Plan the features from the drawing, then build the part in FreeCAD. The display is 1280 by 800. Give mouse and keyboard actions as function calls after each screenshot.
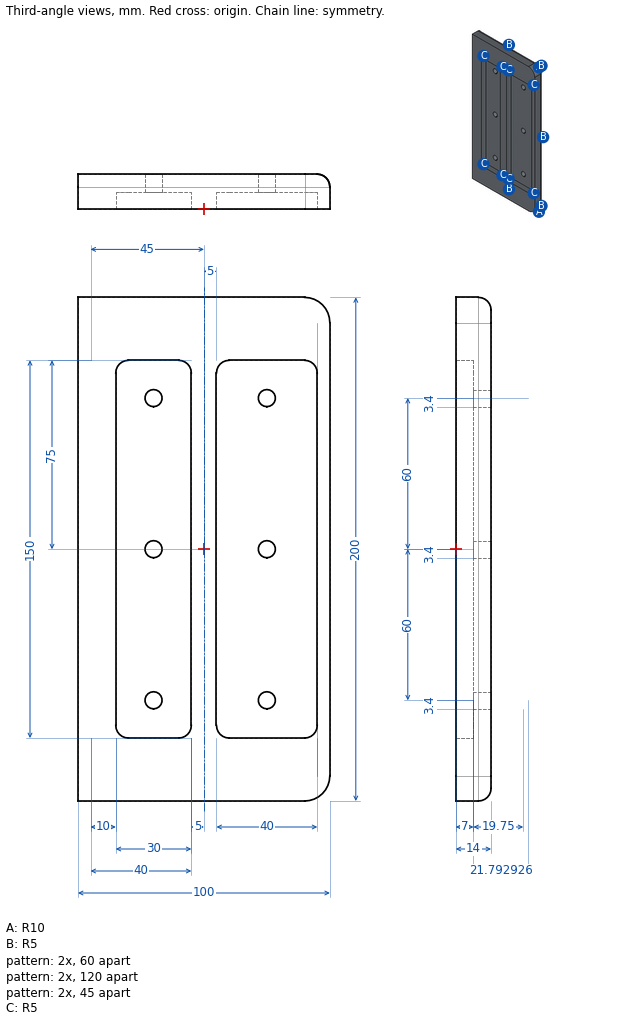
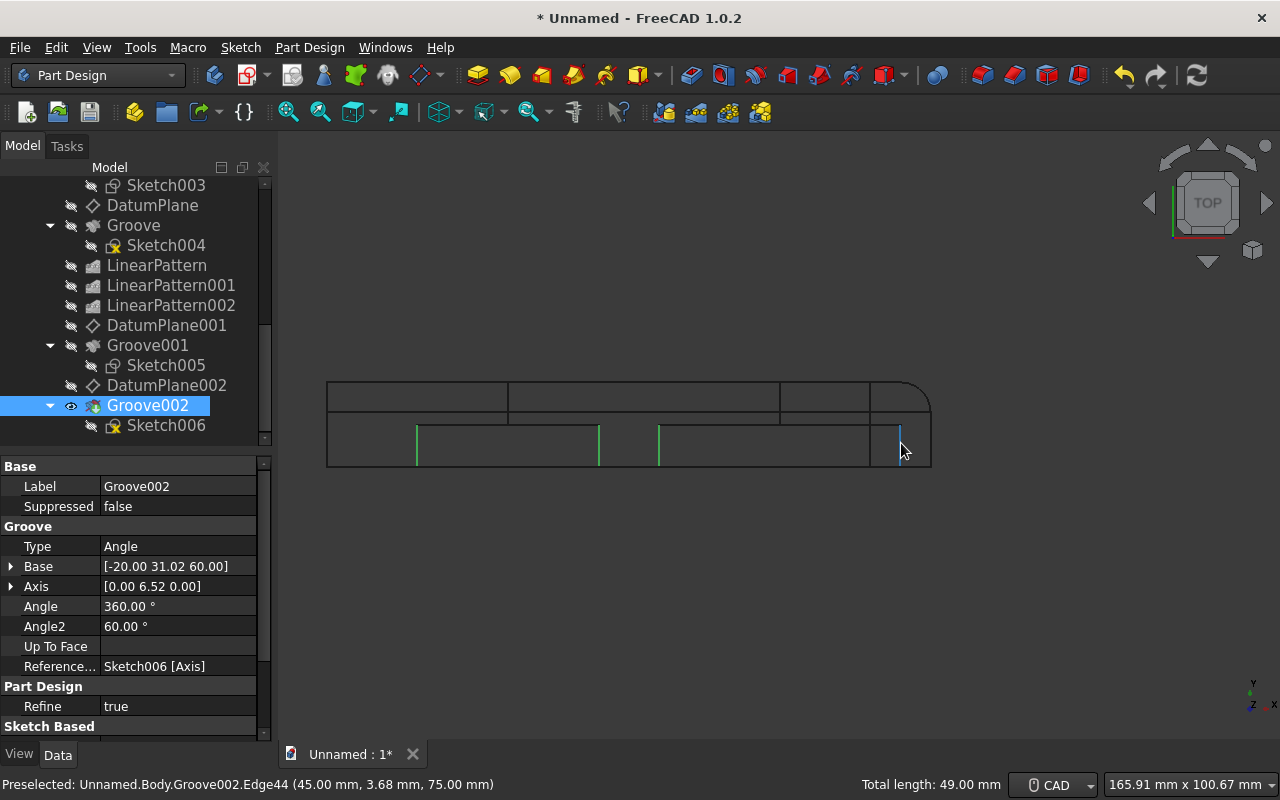
key(v)
key(f)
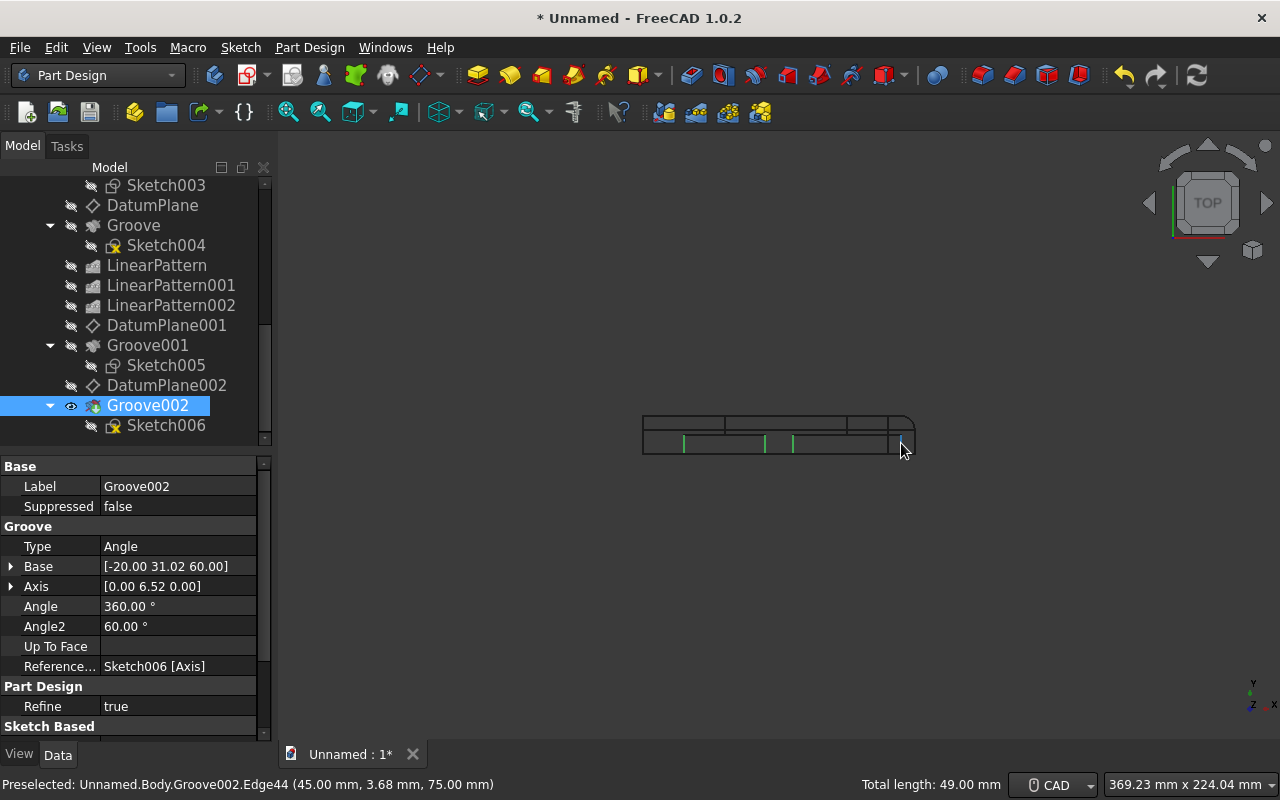
key(1)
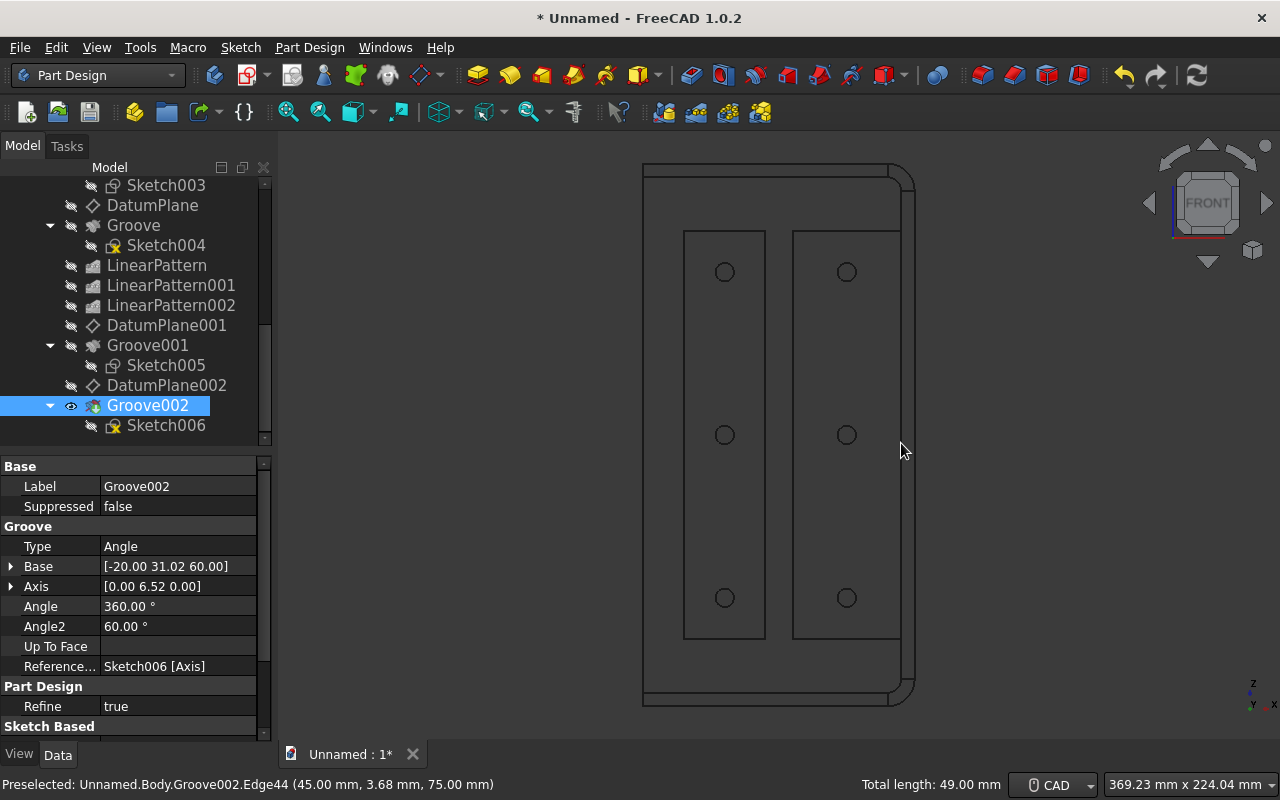
scroll(901, 638, up, 4)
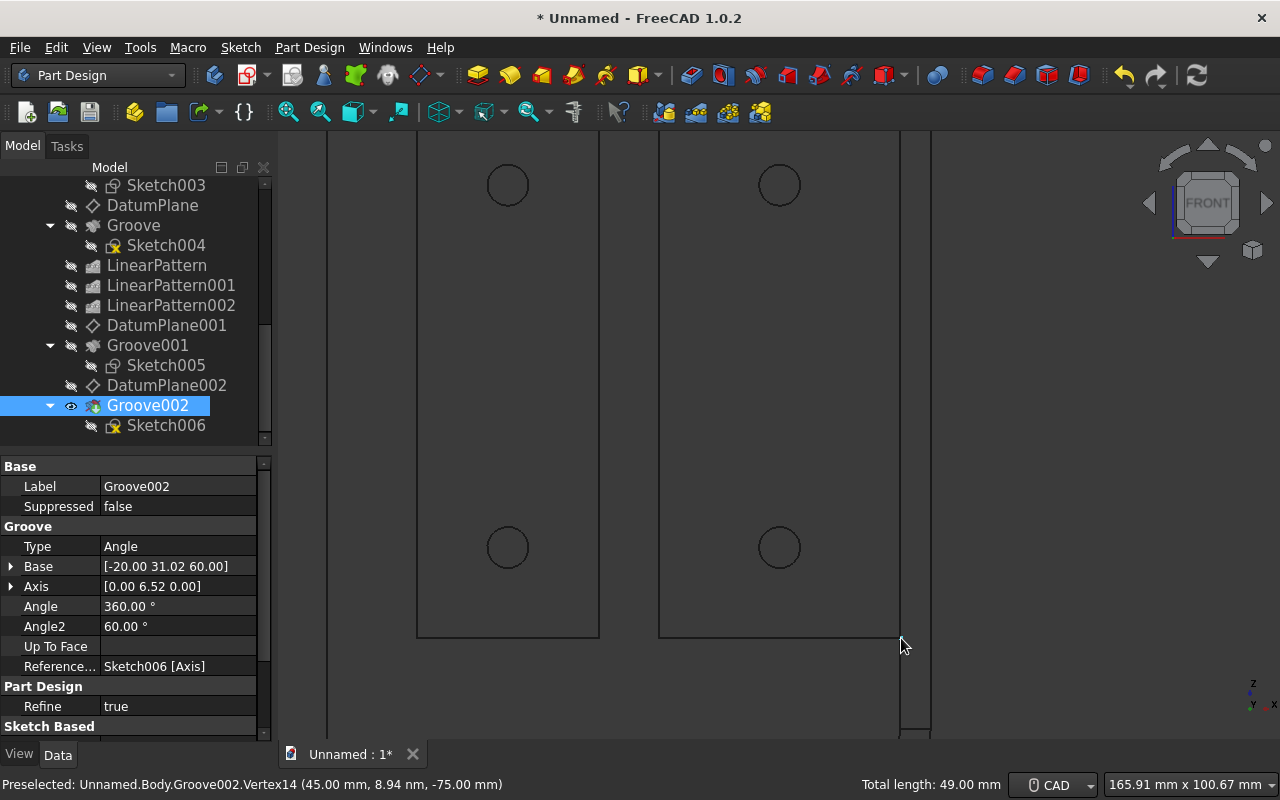
key(v)
key(f)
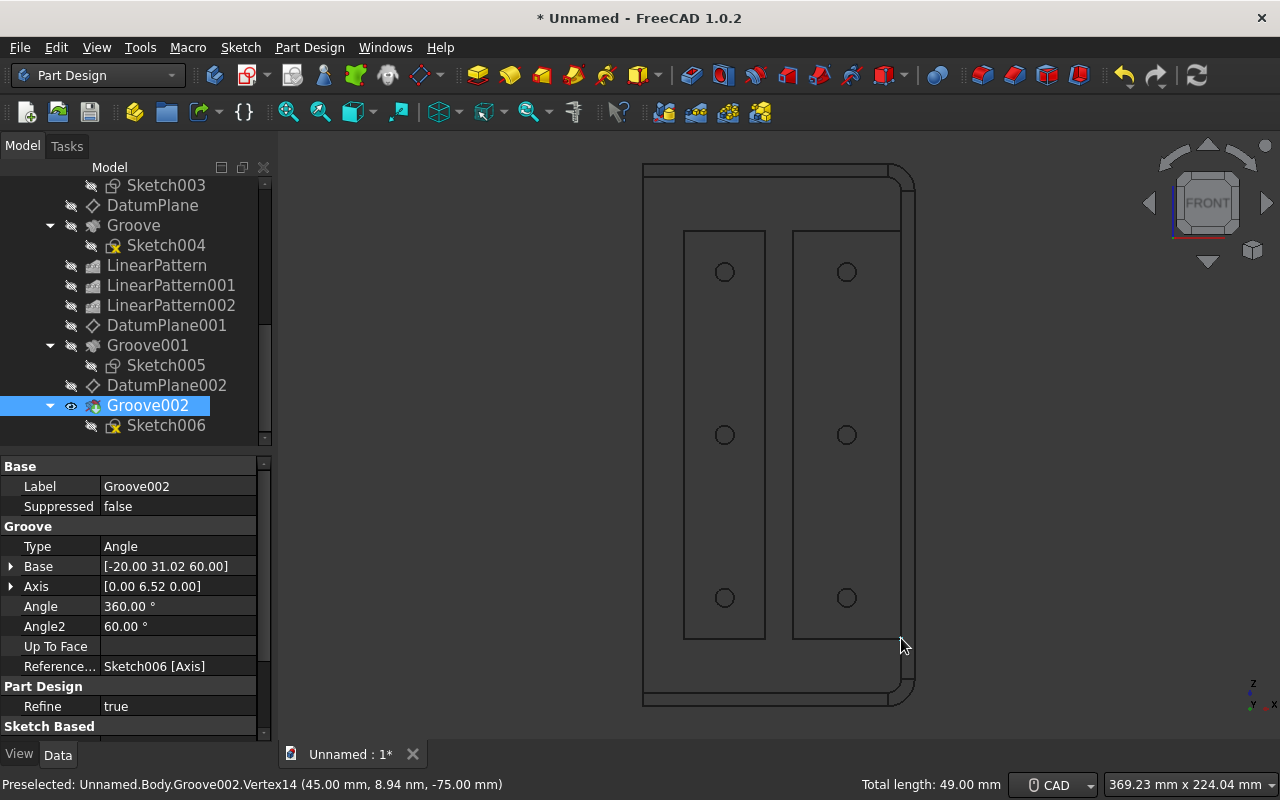
key(3)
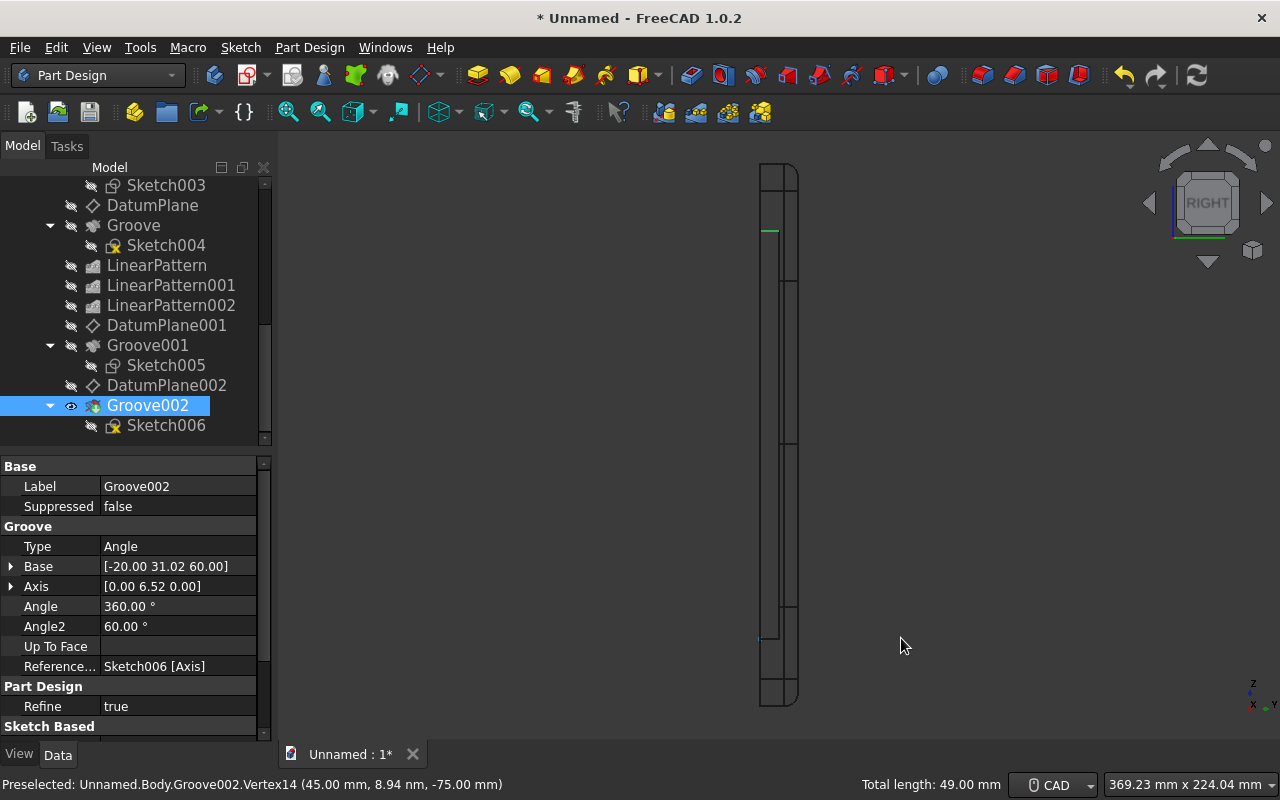
click(770, 638, ctrl)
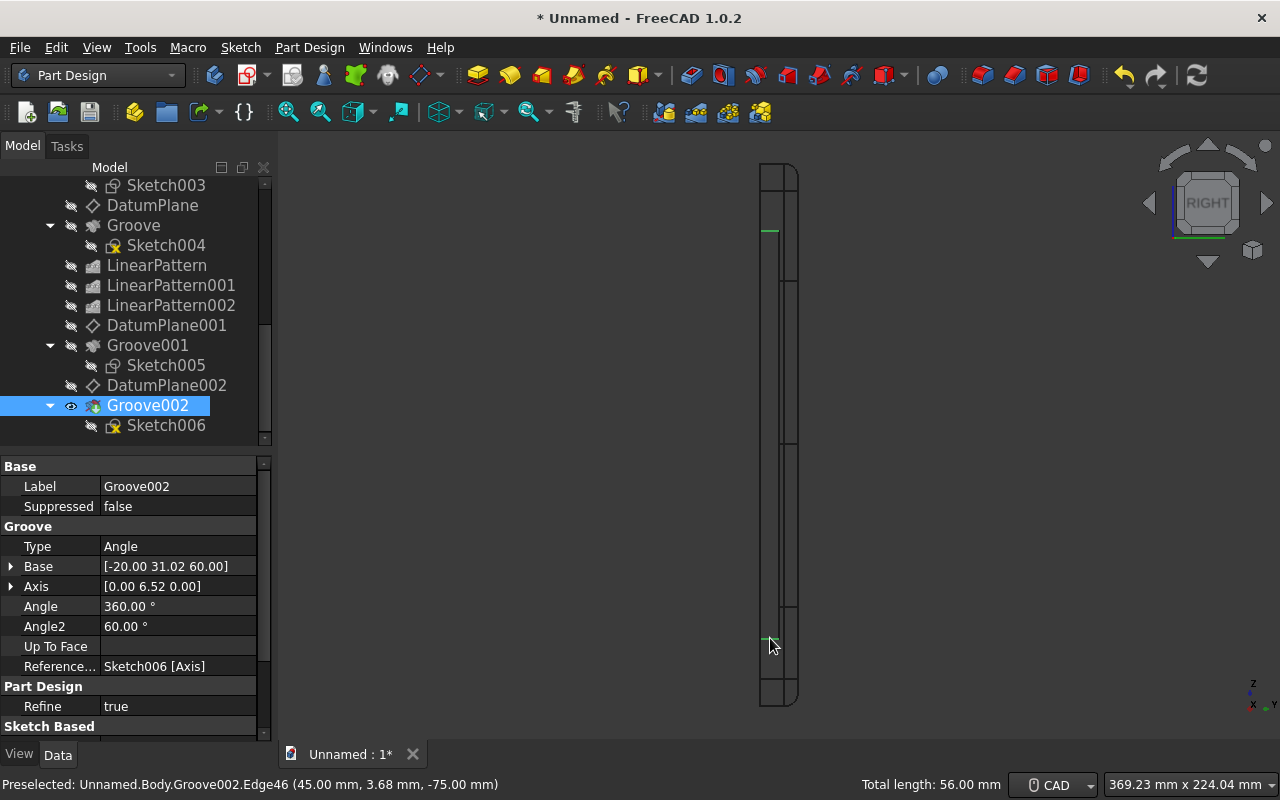
key(v)
key(1)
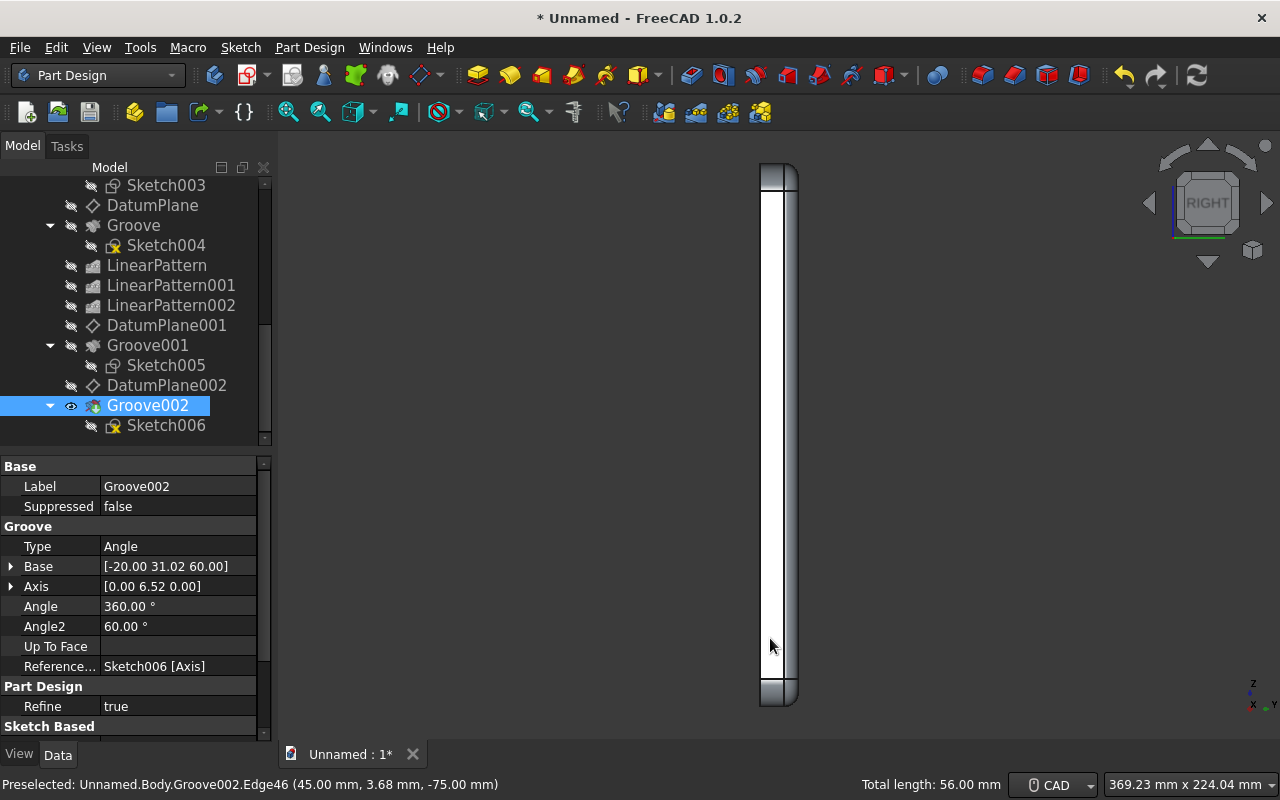
click(984, 76)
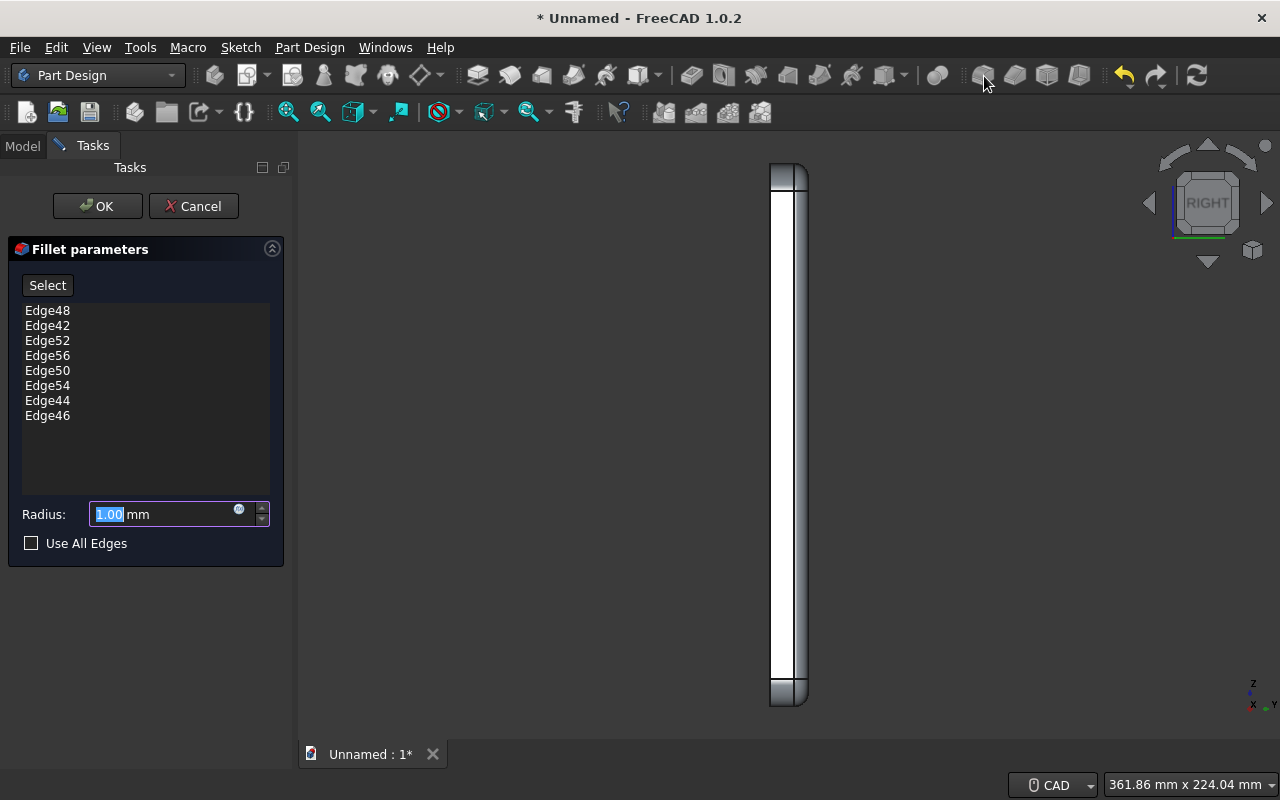
text(5)
key(Tab)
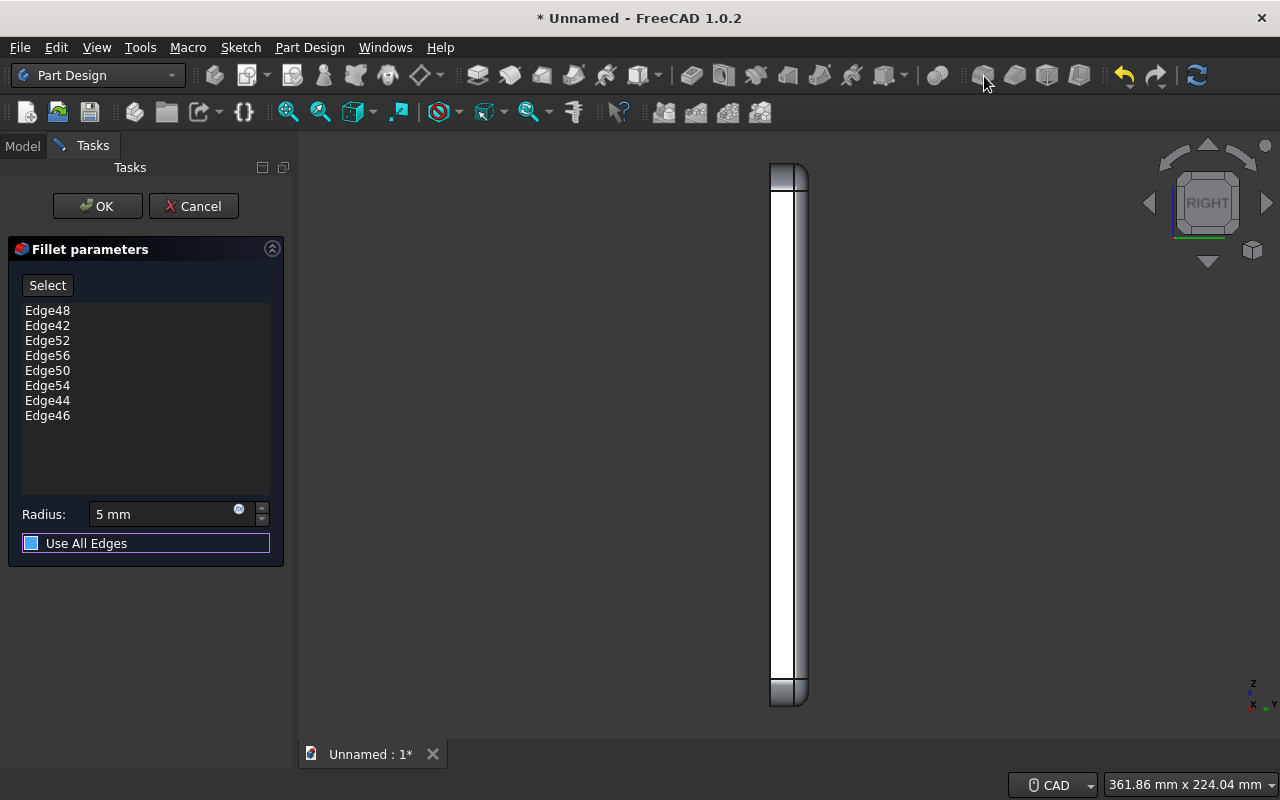
click(98, 206)